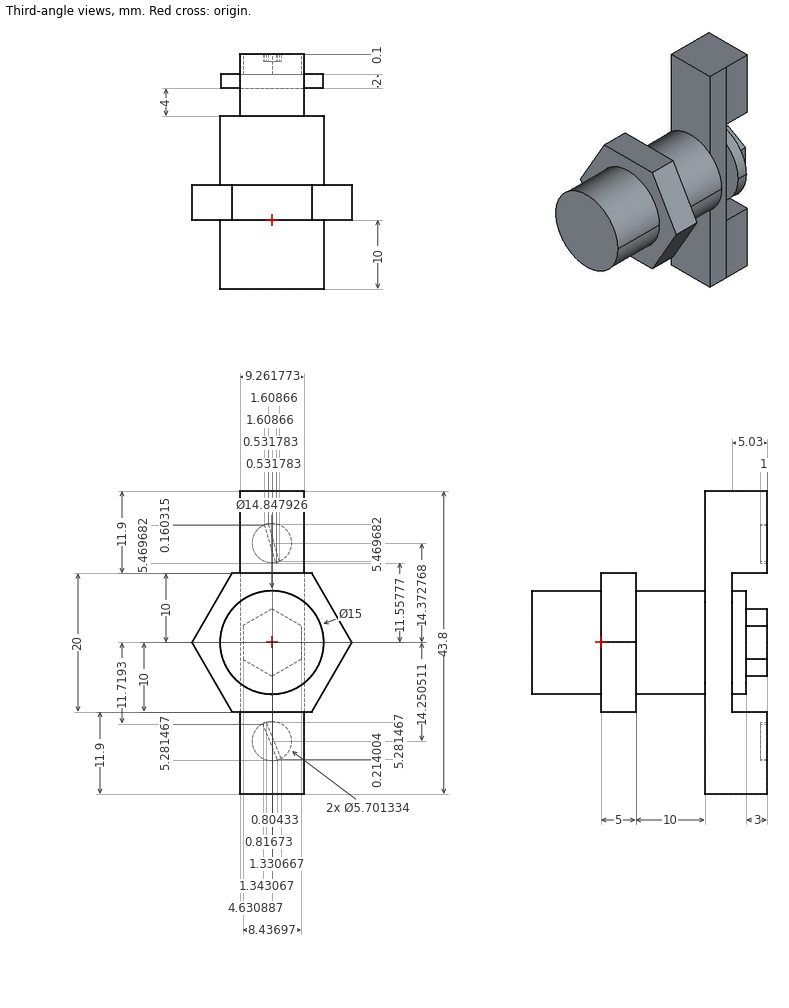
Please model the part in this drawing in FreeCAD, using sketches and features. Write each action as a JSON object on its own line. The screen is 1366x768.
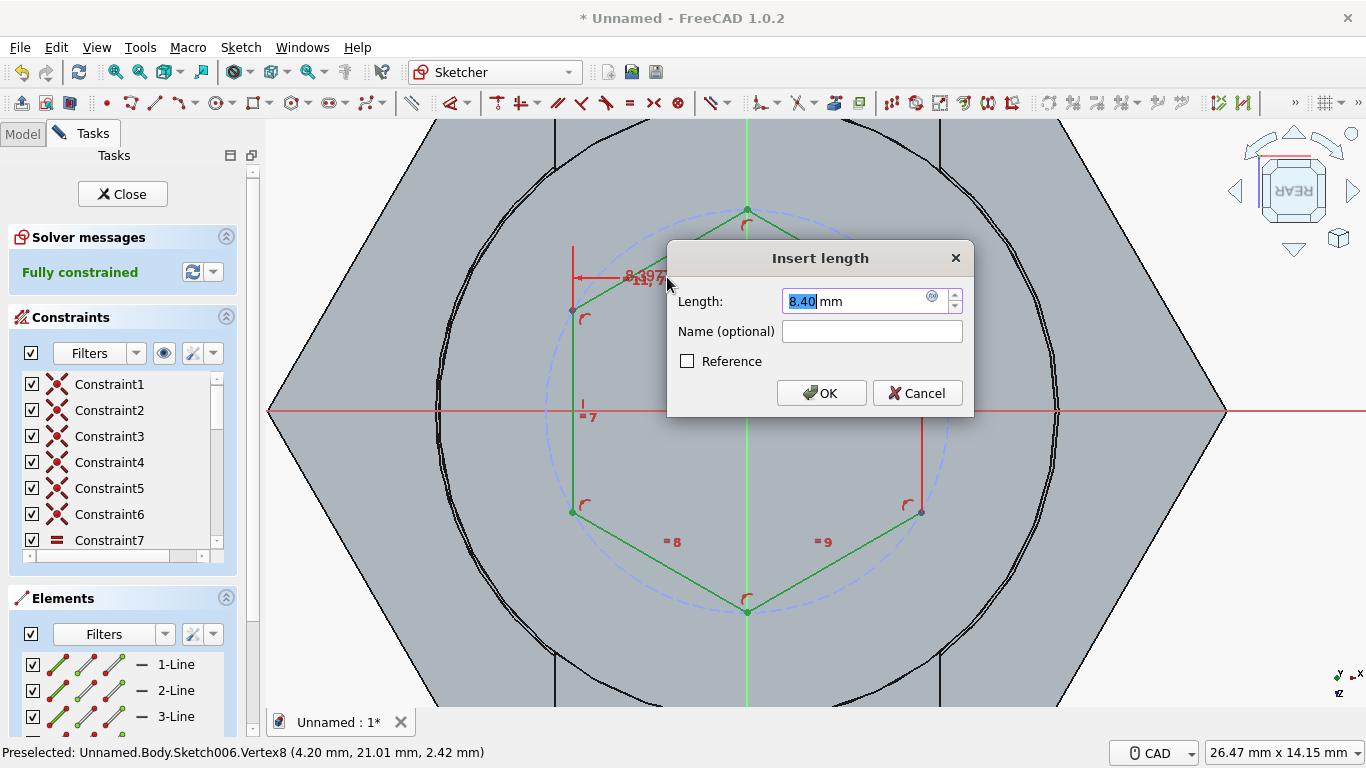
{"action": "type", "text": "8.43697"}
{"action": "key", "text": "Return"}
{"action": "key", "text": "Escape"}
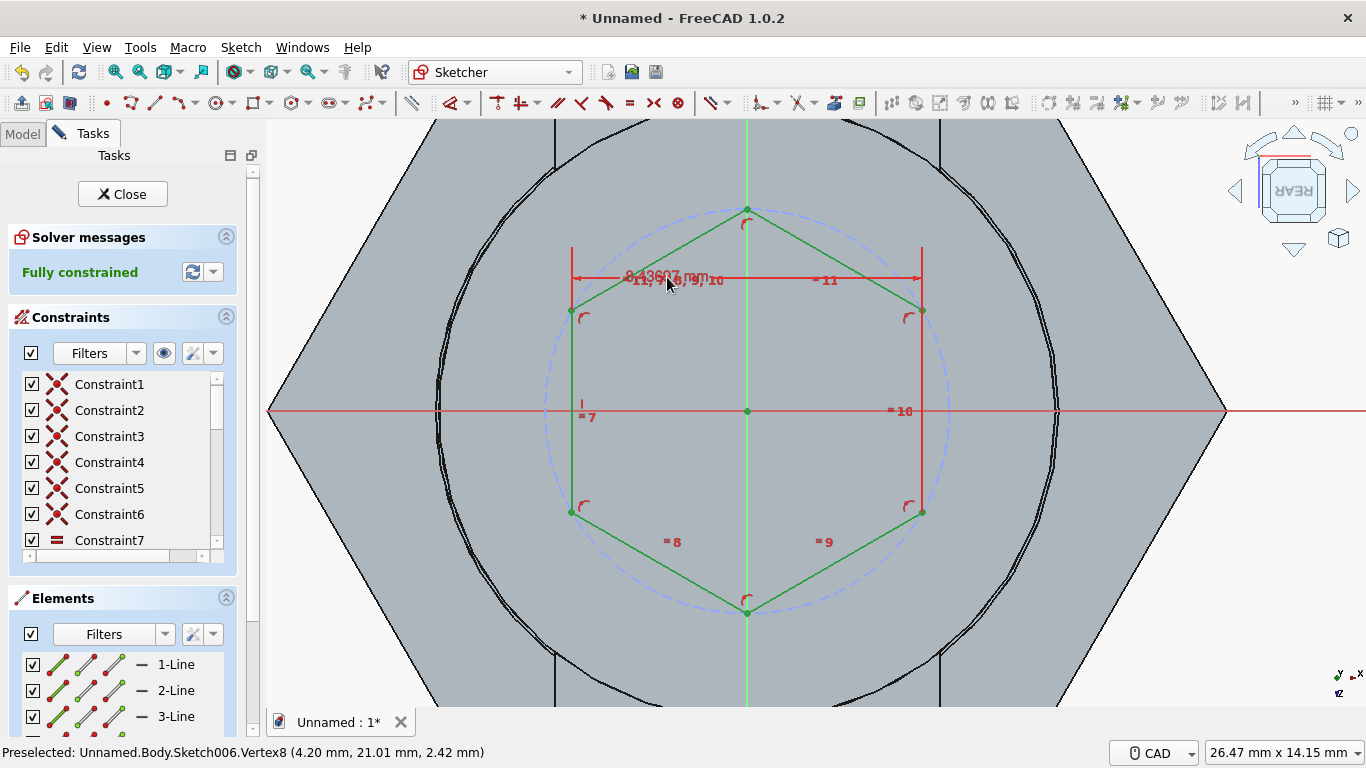
{"action": "left_click", "coordinate": [123, 194]}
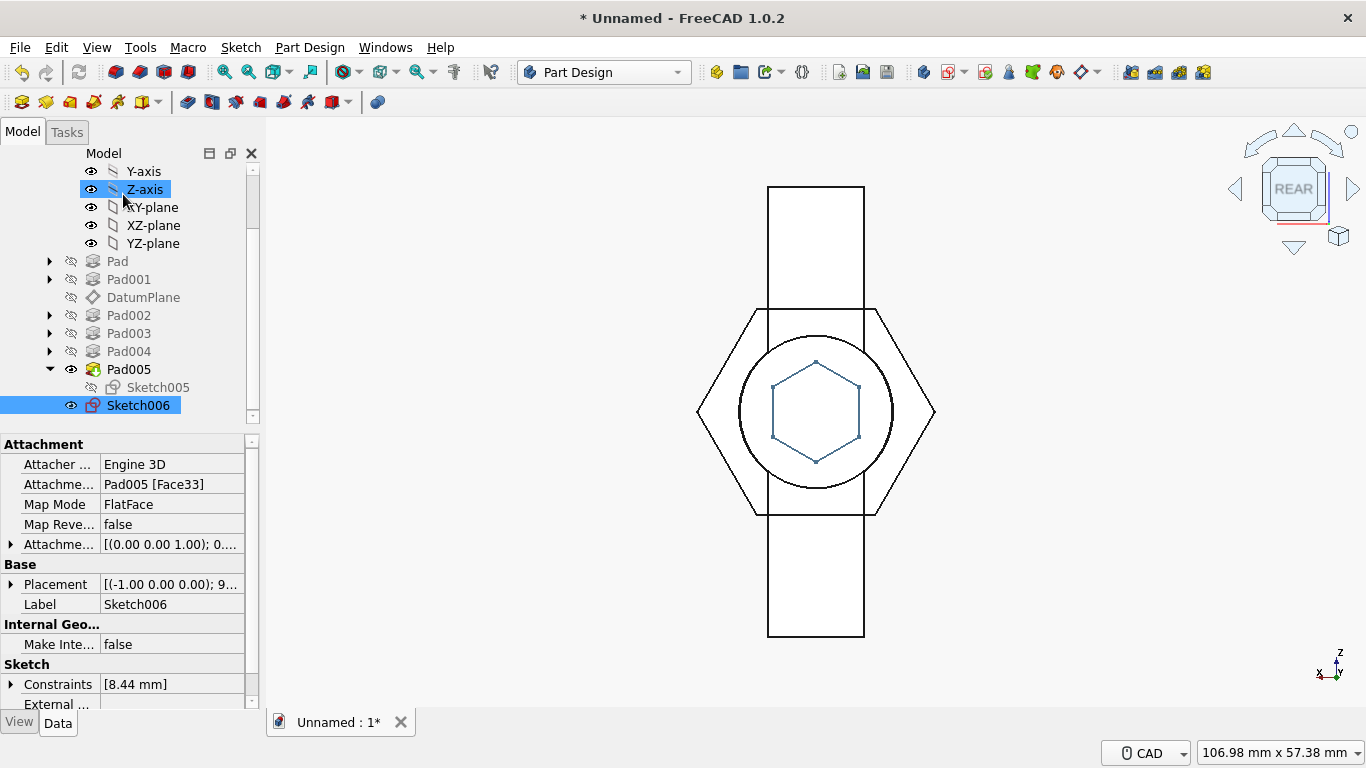
{"action": "left_click", "coordinate": [22, 102]}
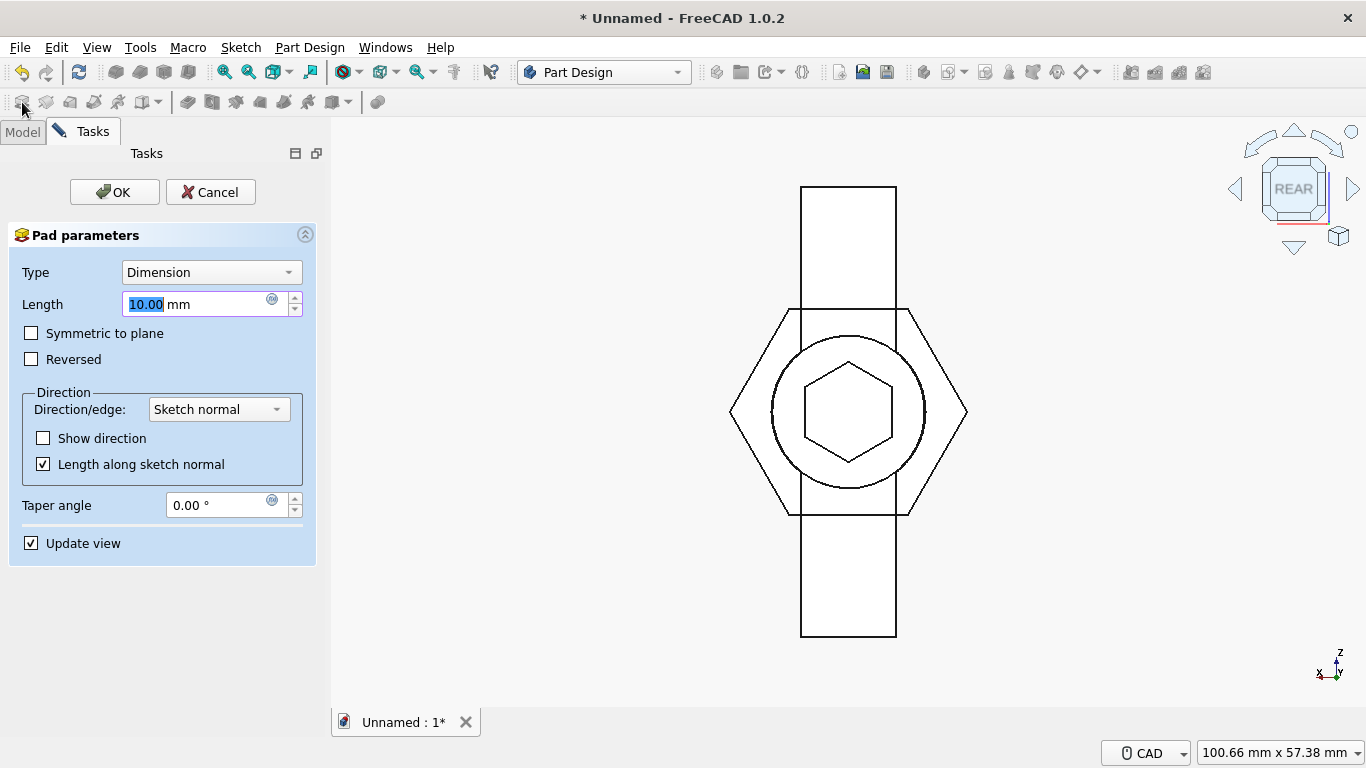
{"action": "type", "text": "3"}
{"action": "key", "text": "Tab"}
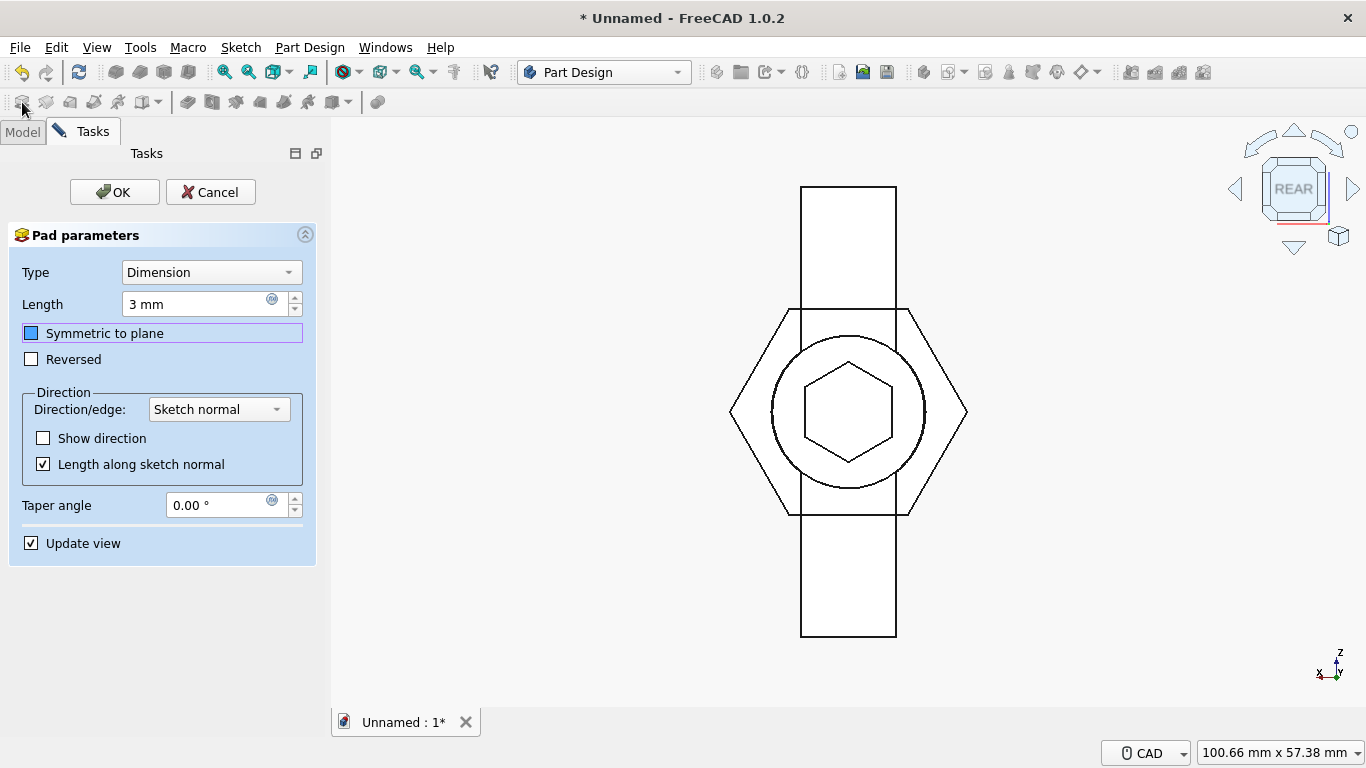
{"action": "left_click", "coordinate": [115, 192]}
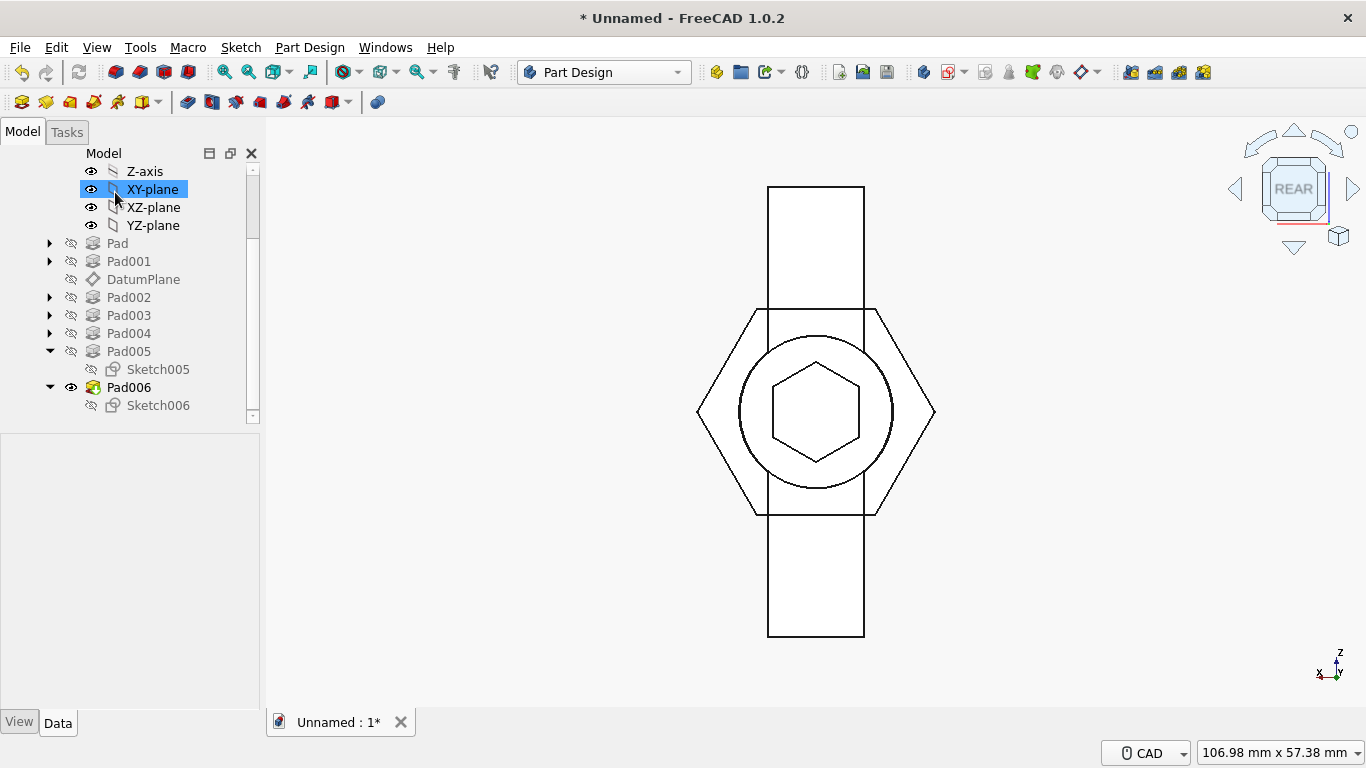
{"action": "left_click", "coordinate": [816, 575]}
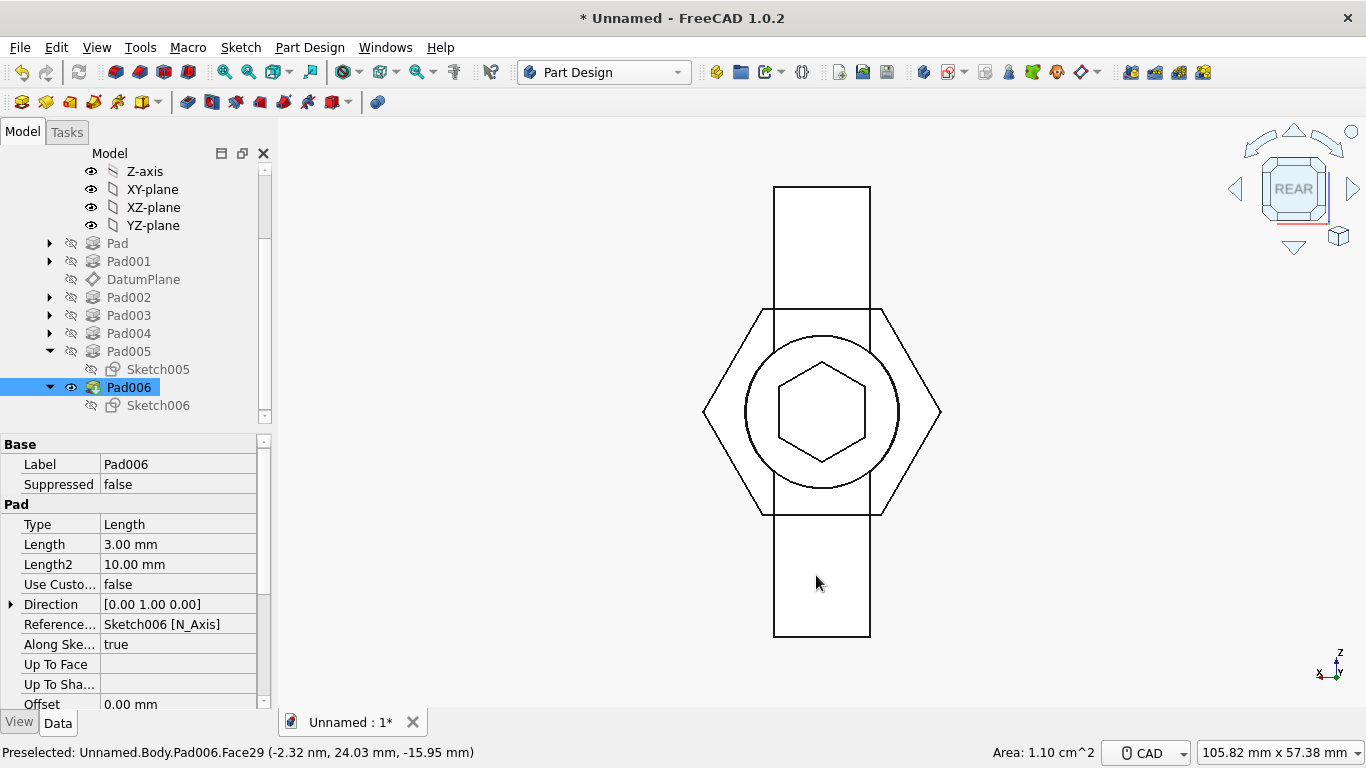
{"action": "left_click", "coordinate": [948, 72]}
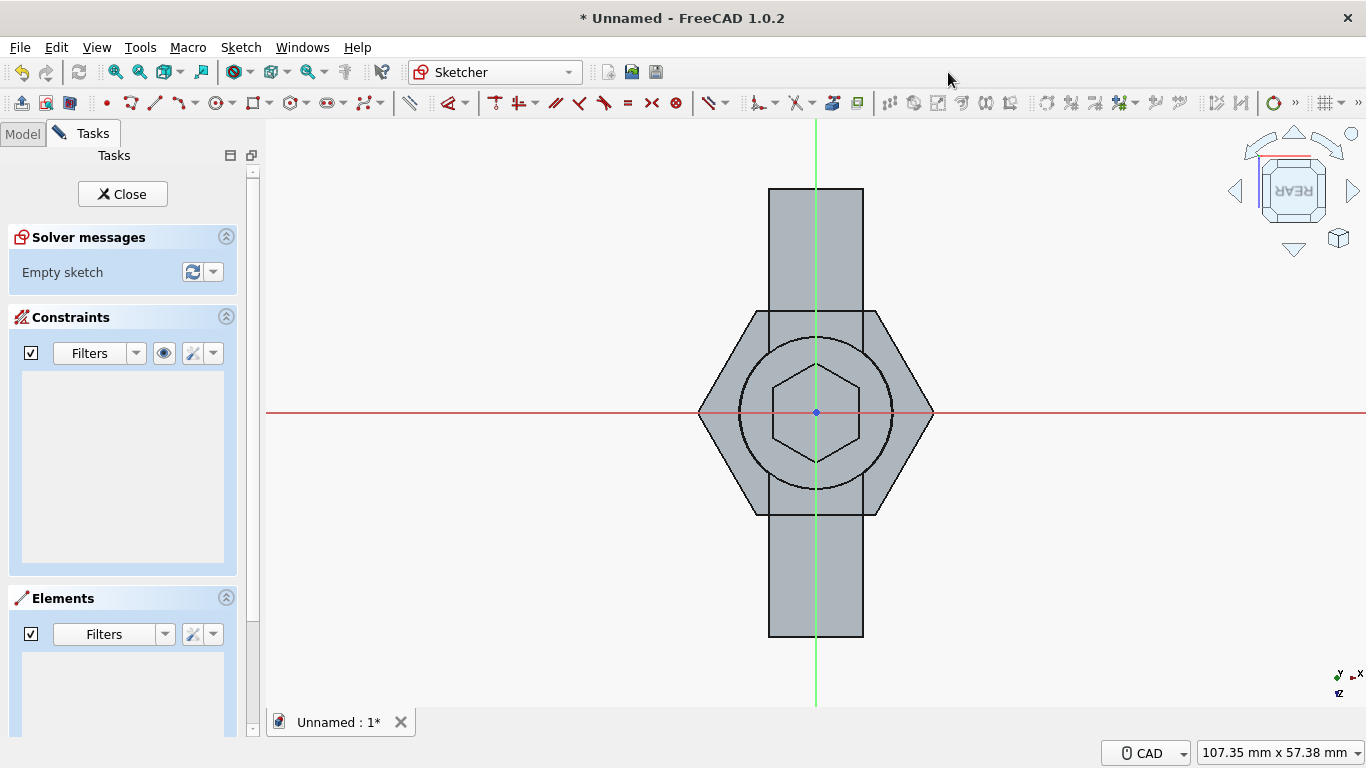
{"action": "left_click", "coordinate": [216, 104]}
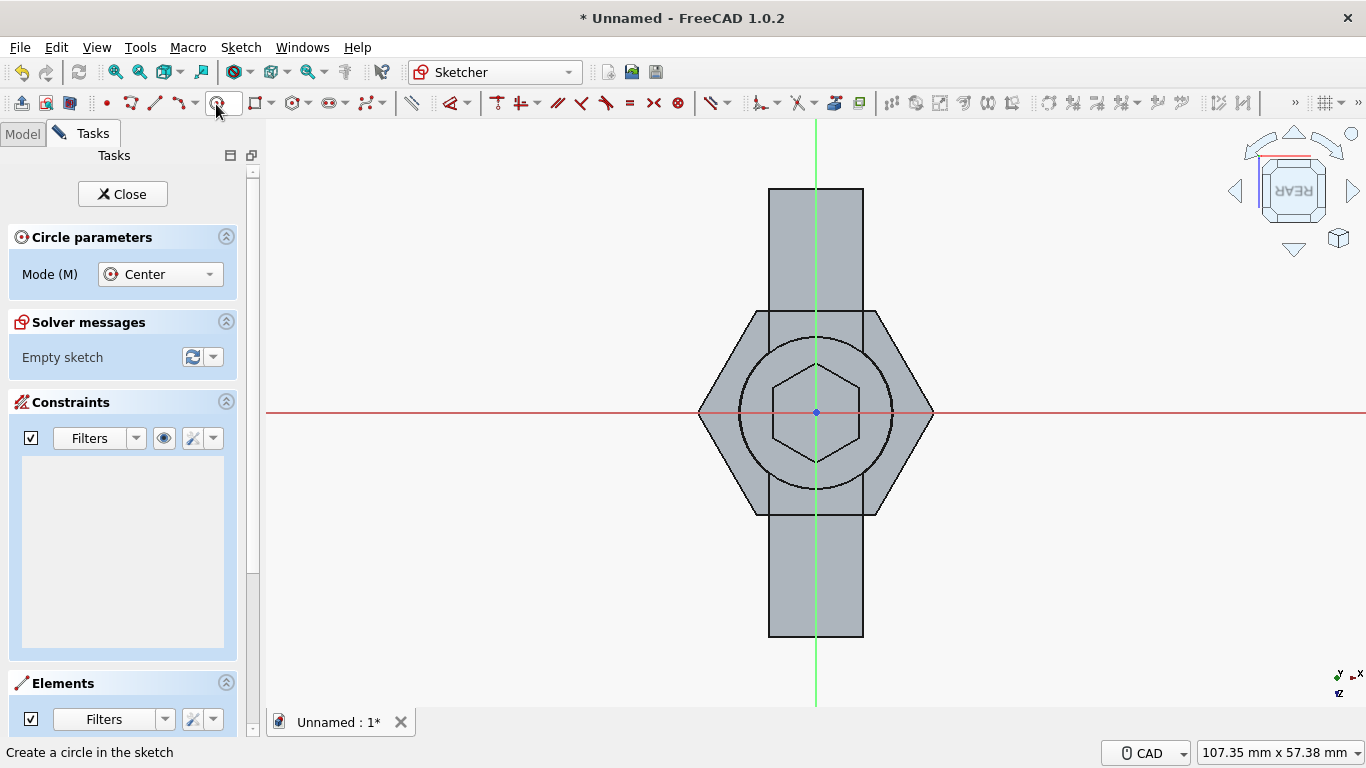
{"action": "left_click", "coordinate": [816, 267]}
{"action": "left_click", "coordinate": [837, 246]}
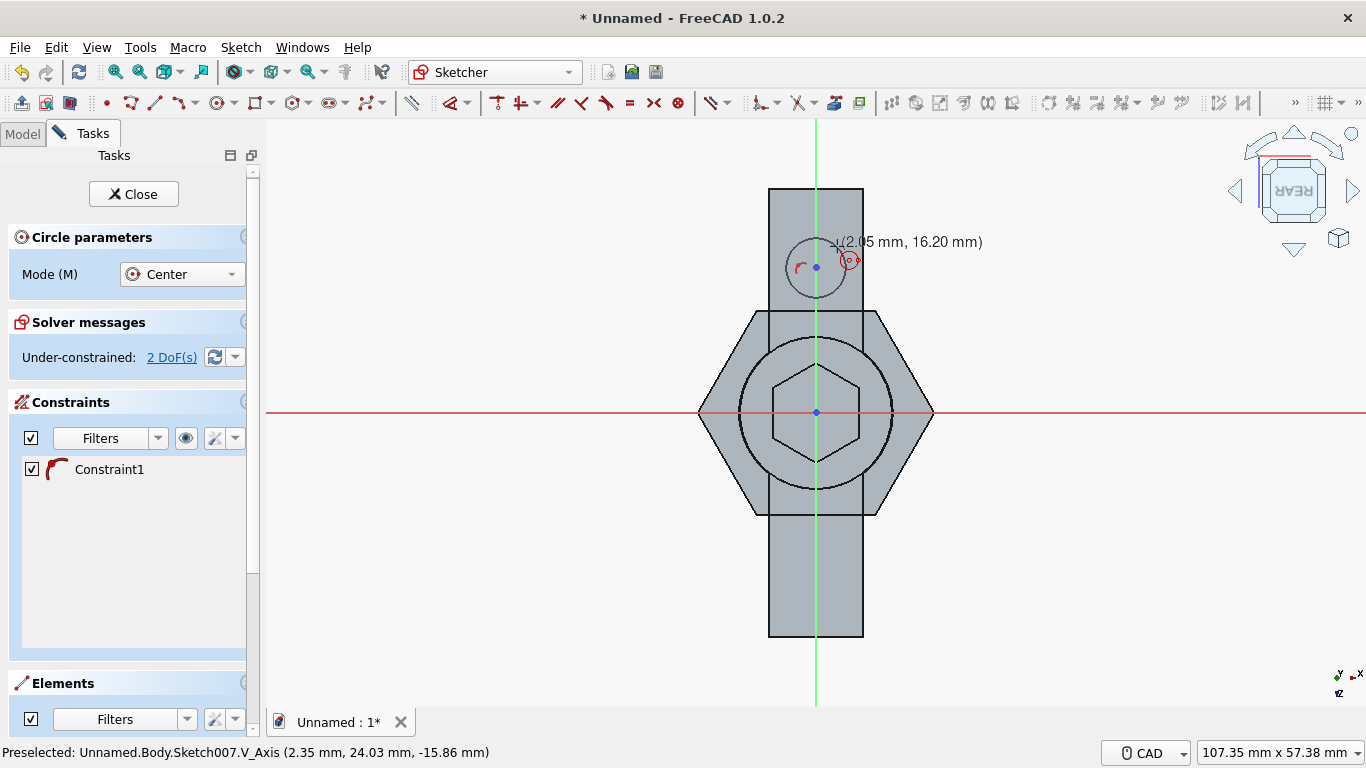
{"action": "left_click", "coordinate": [816, 560]}
{"action": "left_click", "coordinate": [837, 540]}
{"action": "key", "text": "Escape"}